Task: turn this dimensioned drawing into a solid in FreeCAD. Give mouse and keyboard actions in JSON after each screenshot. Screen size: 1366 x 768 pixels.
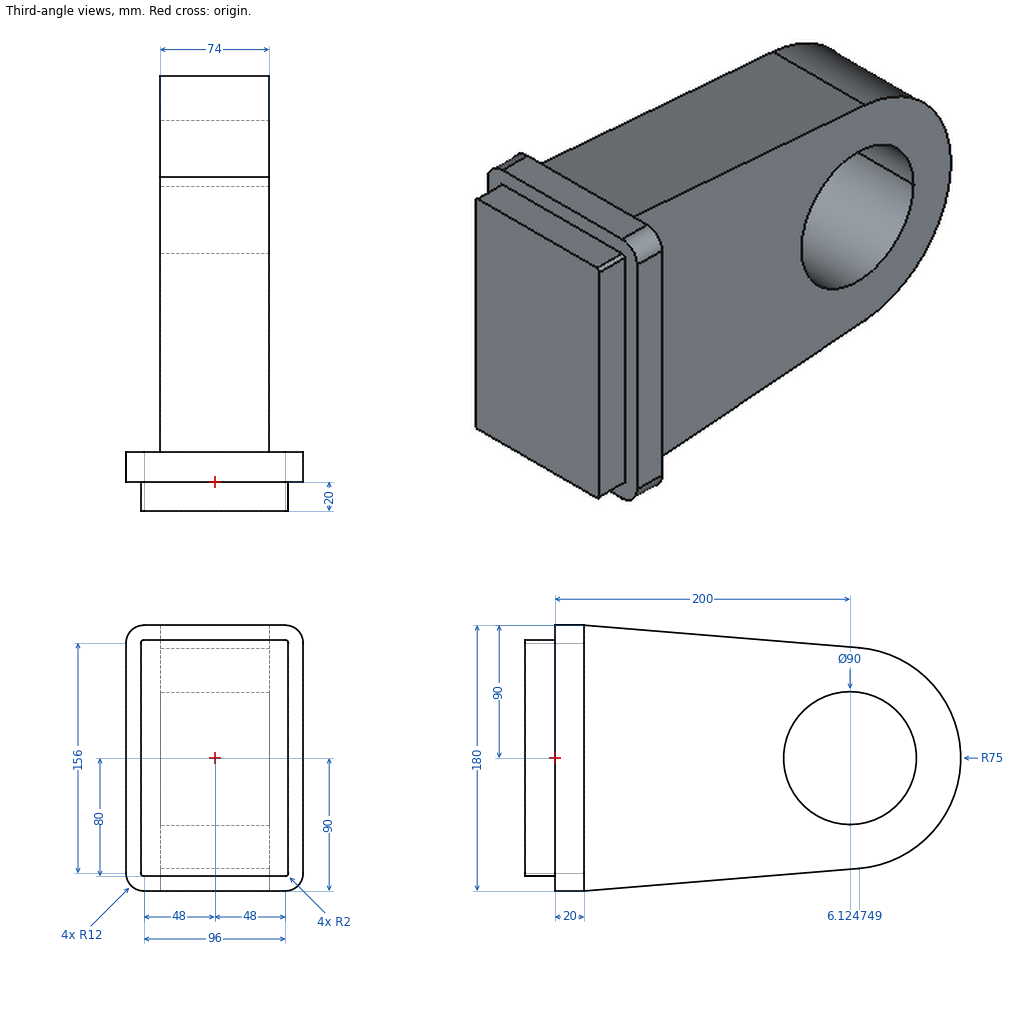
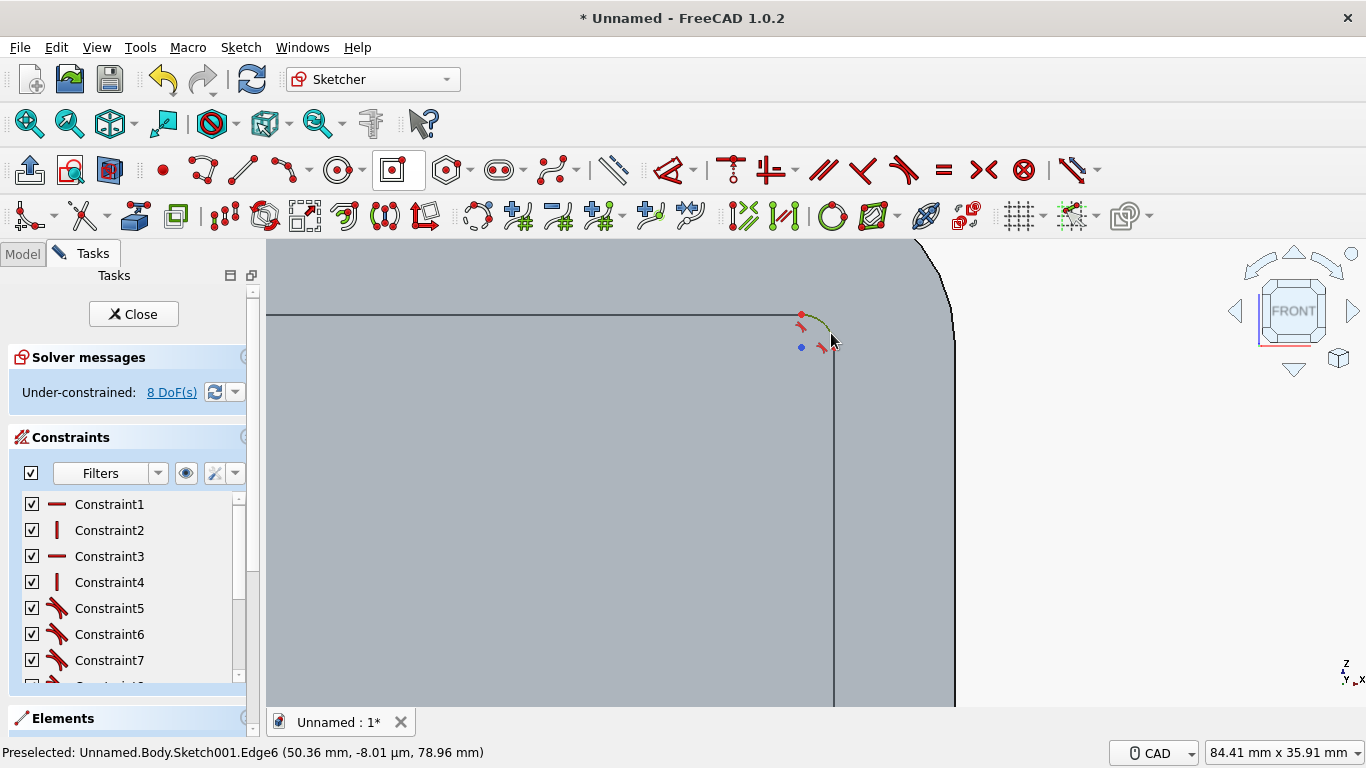
{"action": "scroll", "coordinate": [837, 334], "scroll_direction": "down", "scroll_amount": 10}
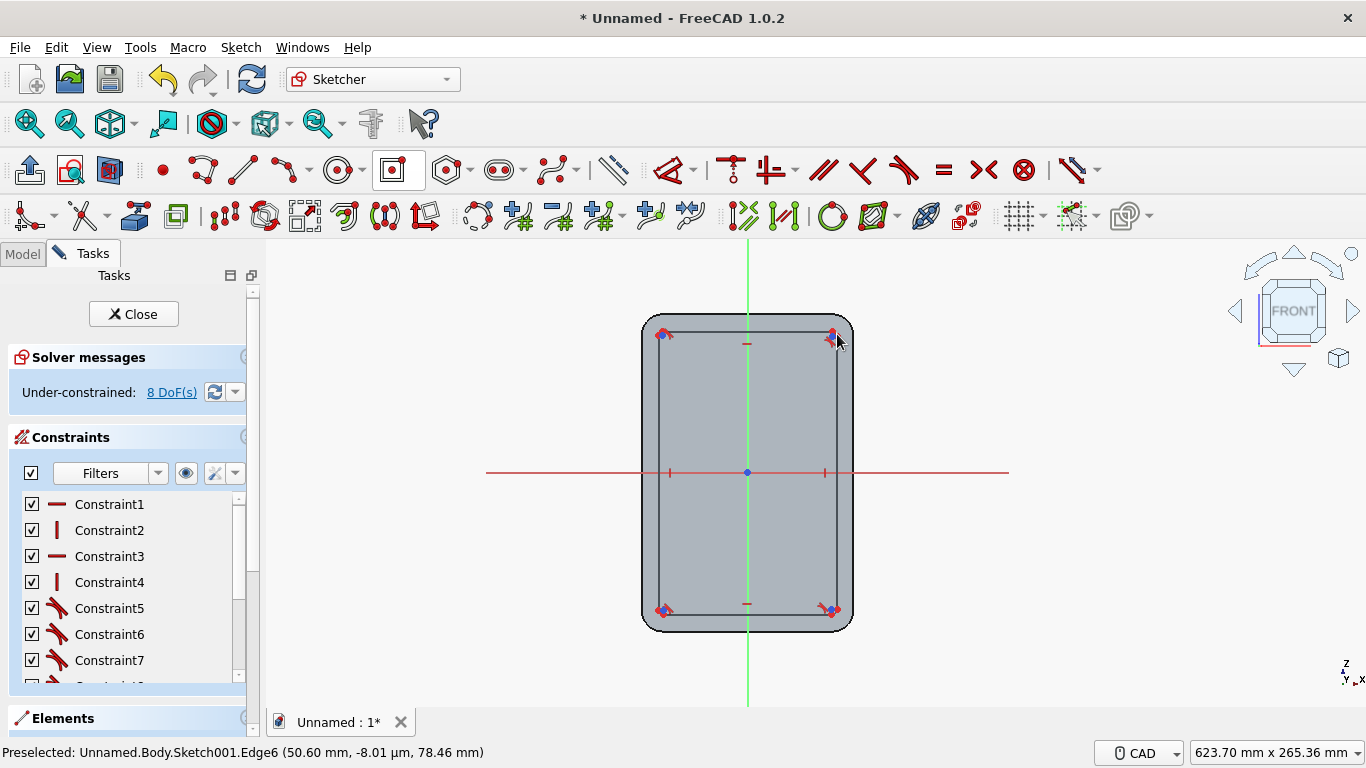
{"action": "scroll", "coordinate": [661, 332], "scroll_direction": "up", "scroll_amount": 10}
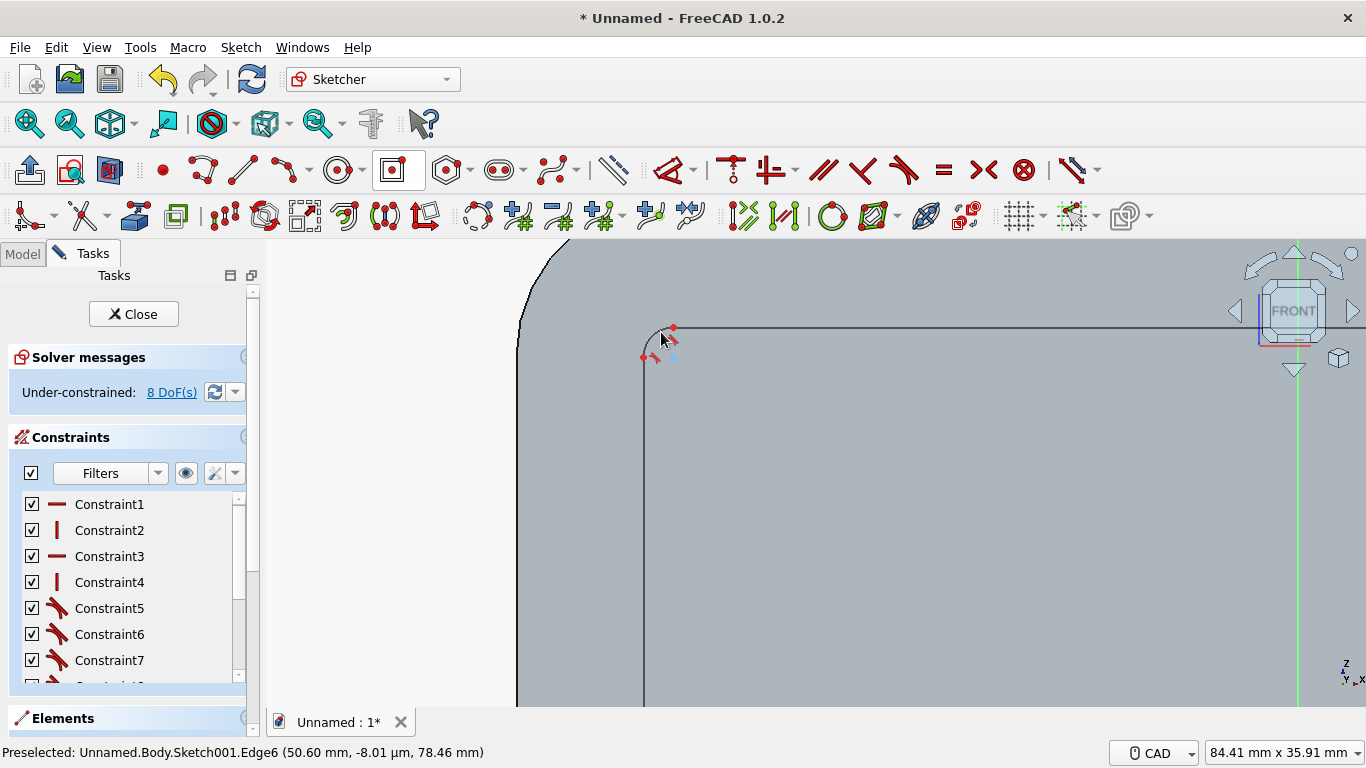
{"action": "left_click", "coordinate": [660, 331]}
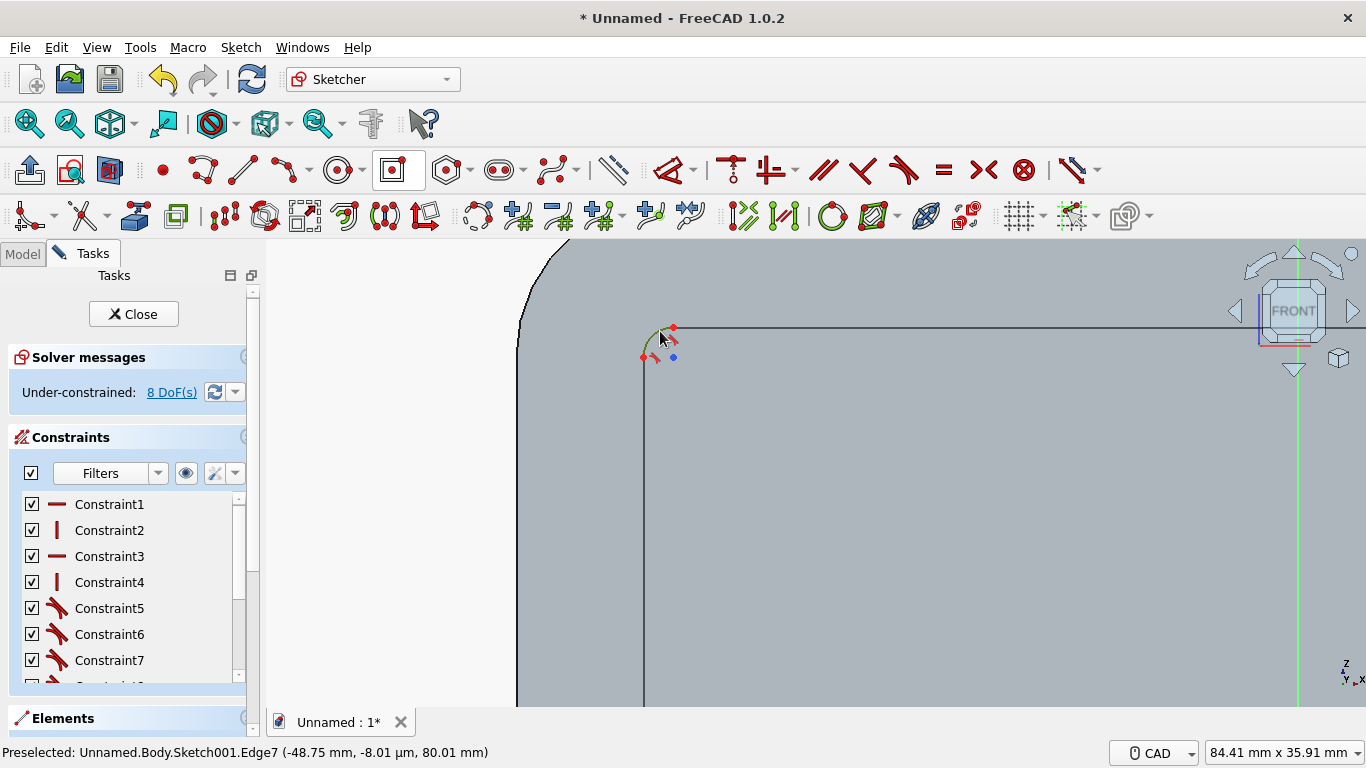
{"action": "scroll", "coordinate": [661, 332], "scroll_direction": "down", "scroll_amount": 10}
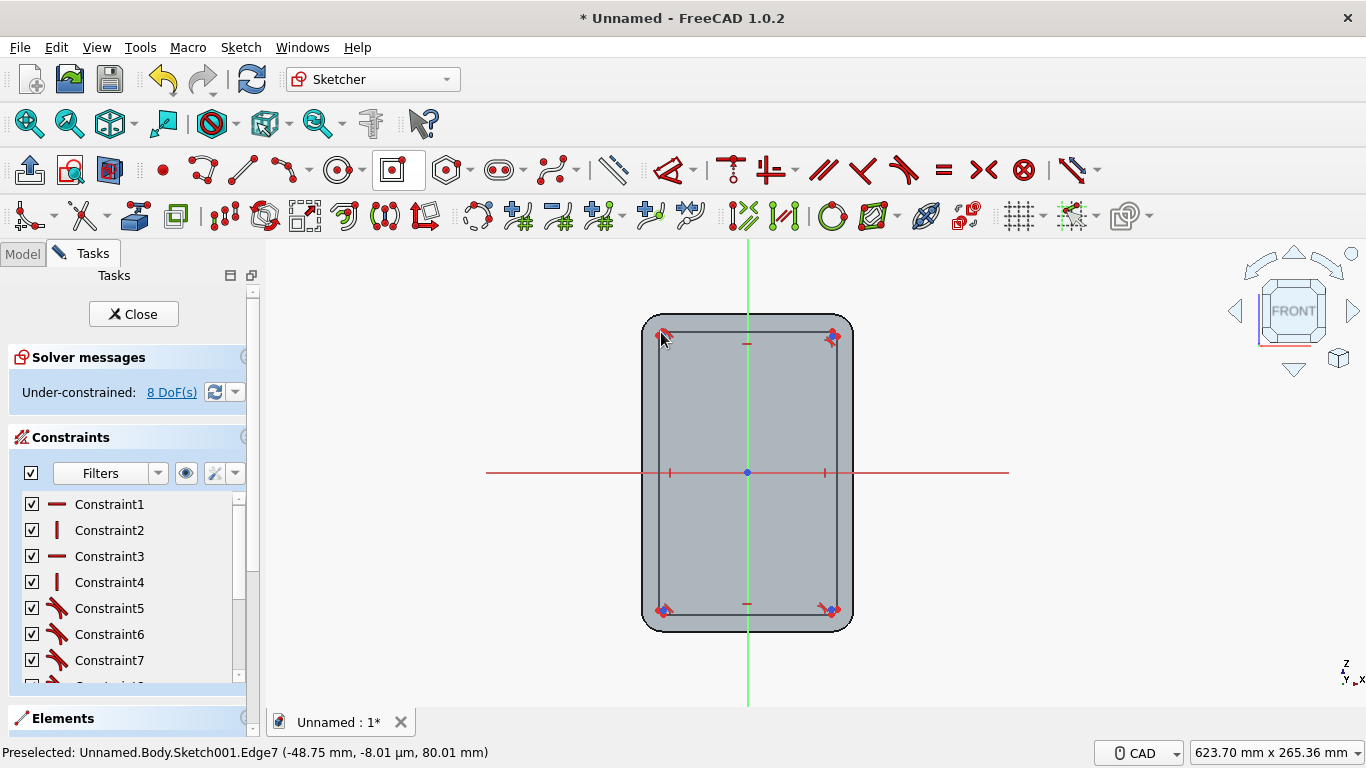
{"action": "scroll", "coordinate": [659, 612], "scroll_direction": "up", "scroll_amount": 10}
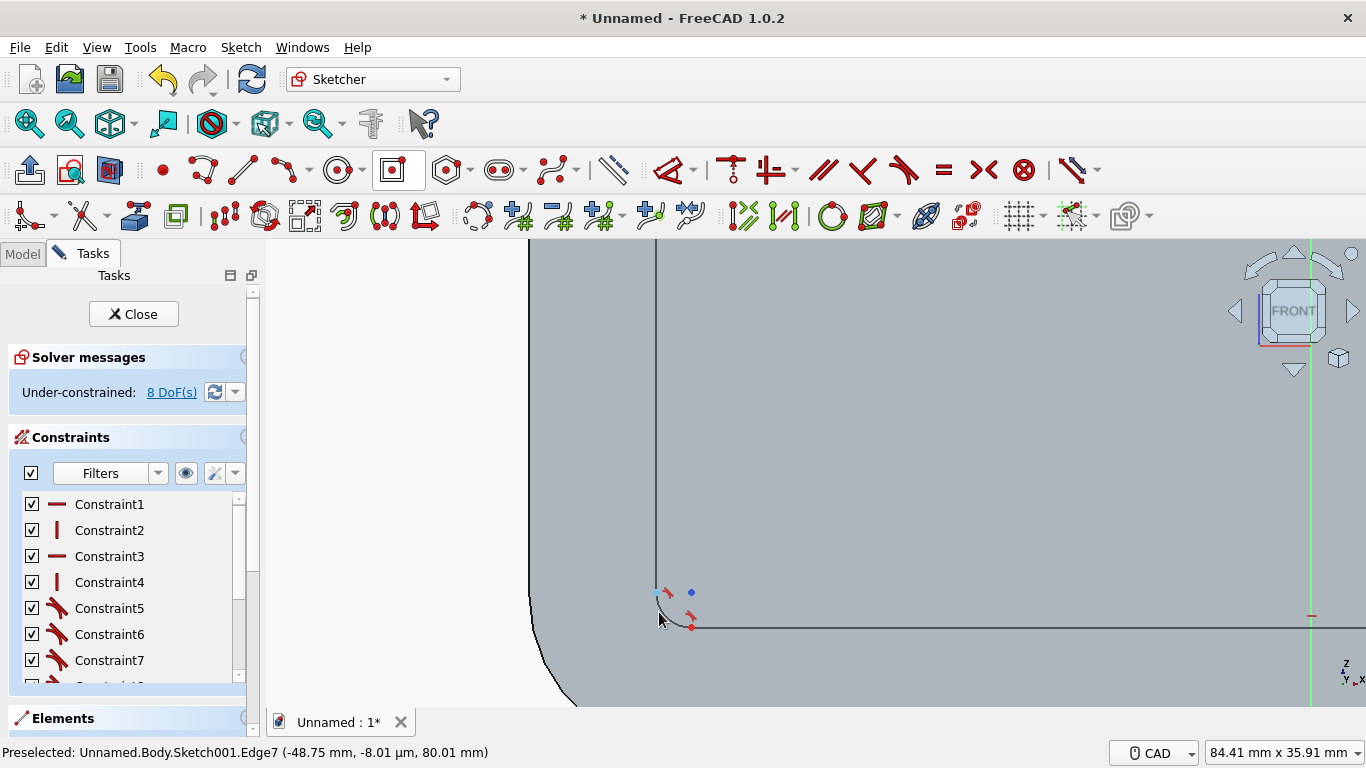
{"action": "left_click", "coordinate": [660, 608]}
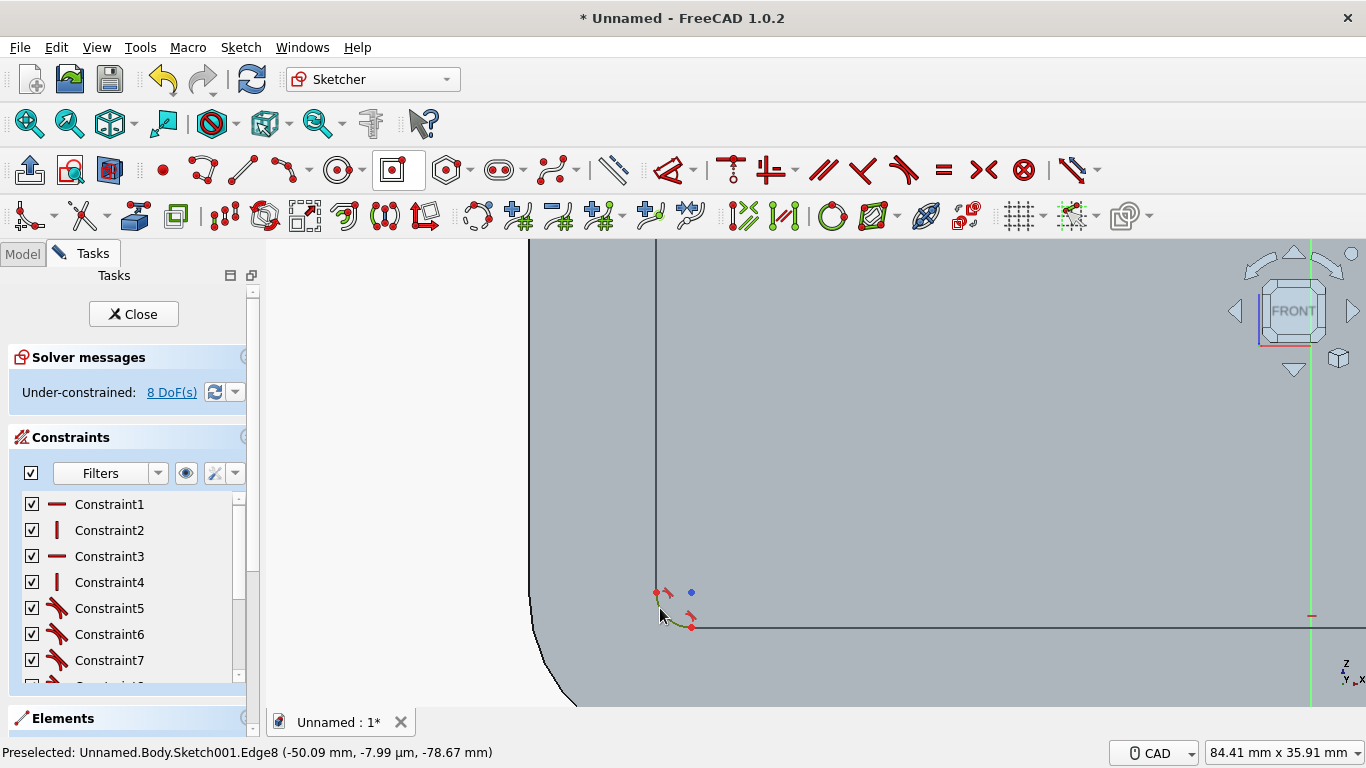
{"action": "key", "text": "e"}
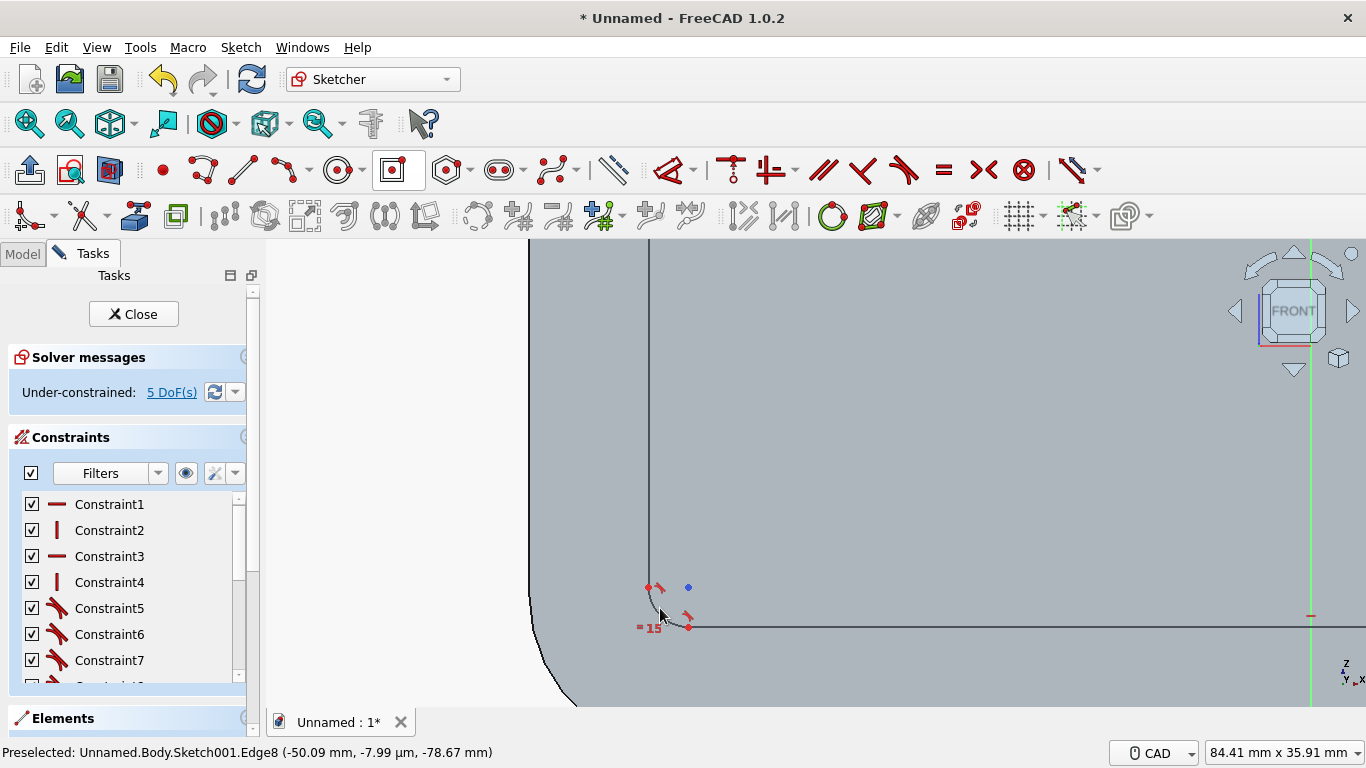
{"action": "left_click", "coordinate": [668, 170]}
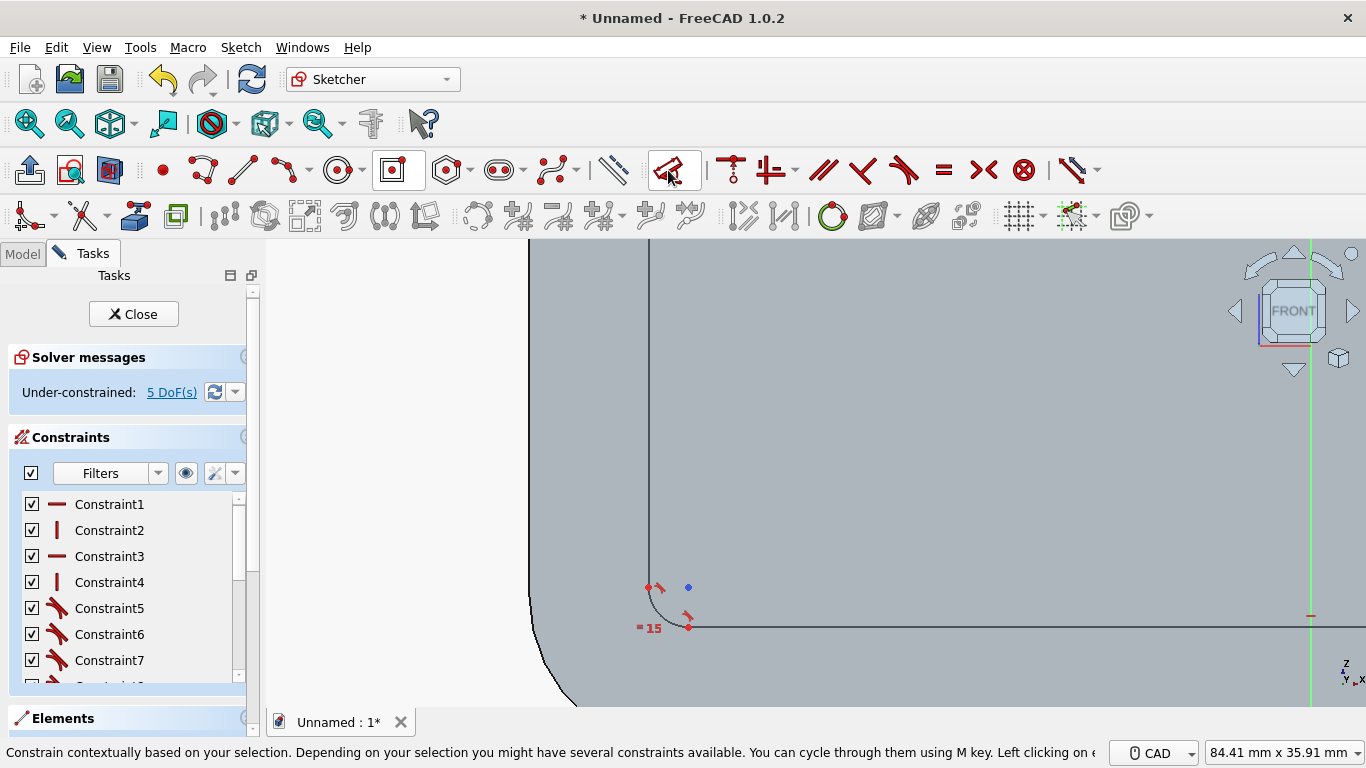
{"action": "scroll", "coordinate": [659, 613], "scroll_direction": "down", "scroll_amount": 10}